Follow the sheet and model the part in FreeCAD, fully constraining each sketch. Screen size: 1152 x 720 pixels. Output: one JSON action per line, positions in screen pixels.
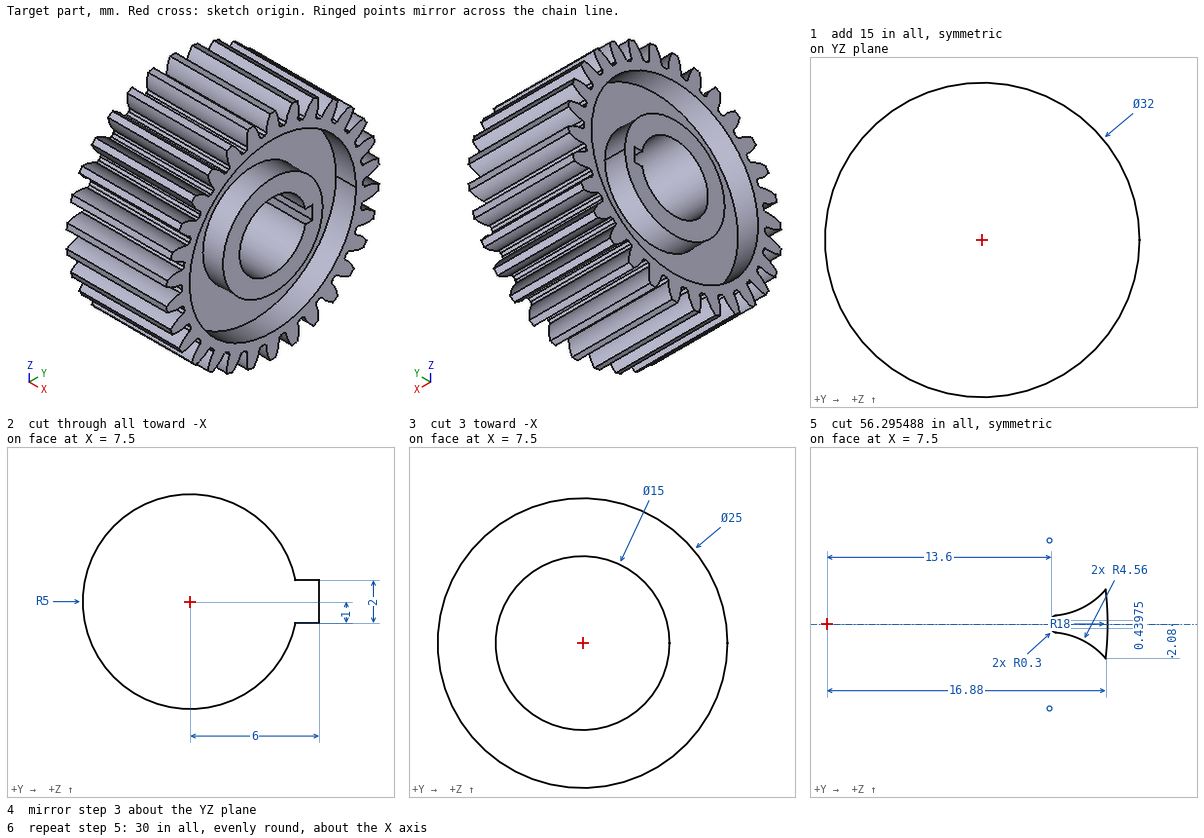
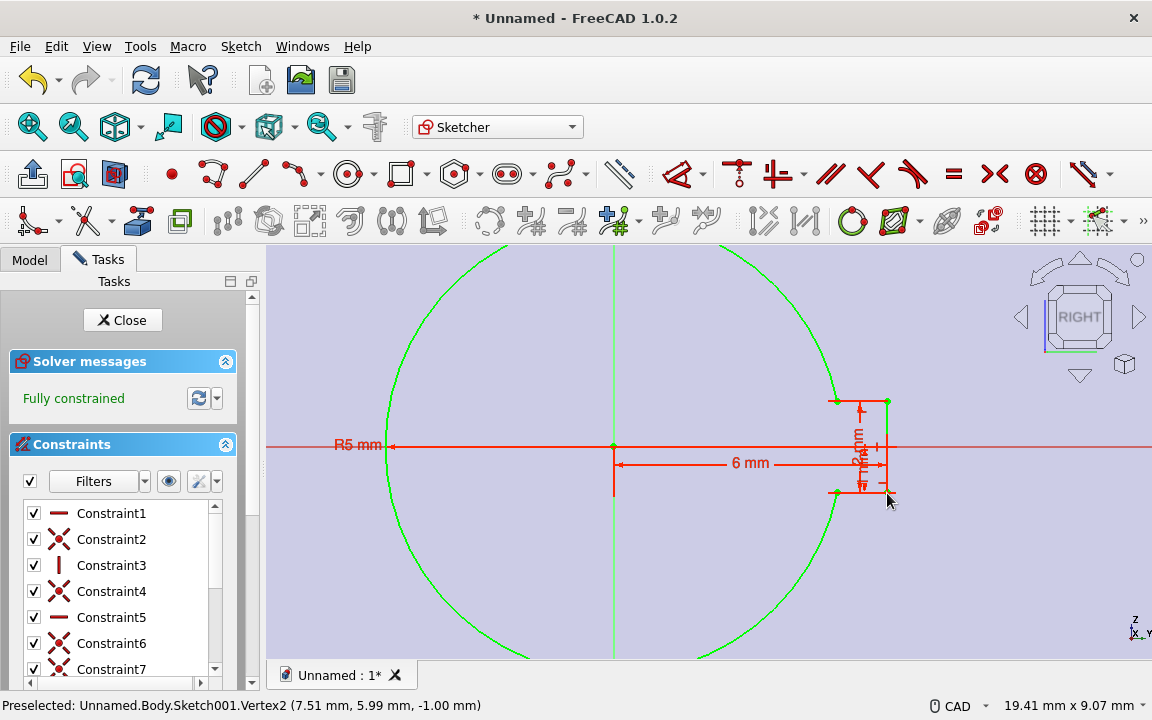
{"action": "left_click", "coordinate": [123, 320]}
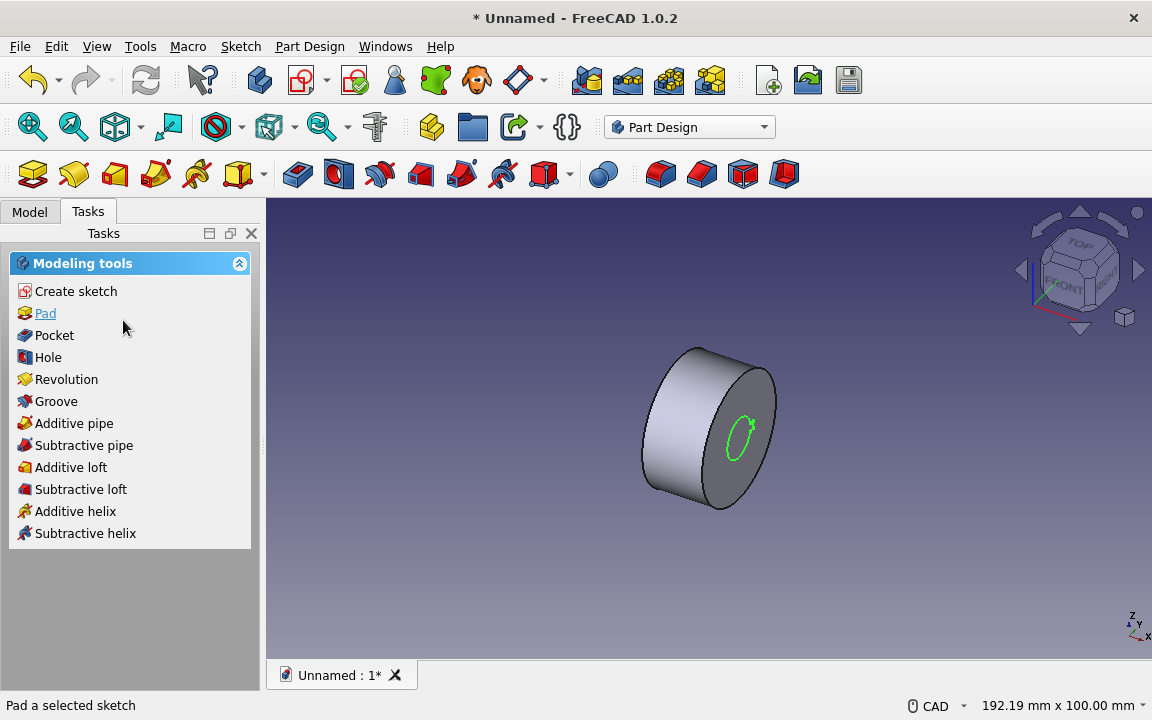
{"action": "left_click", "coordinate": [298, 174]}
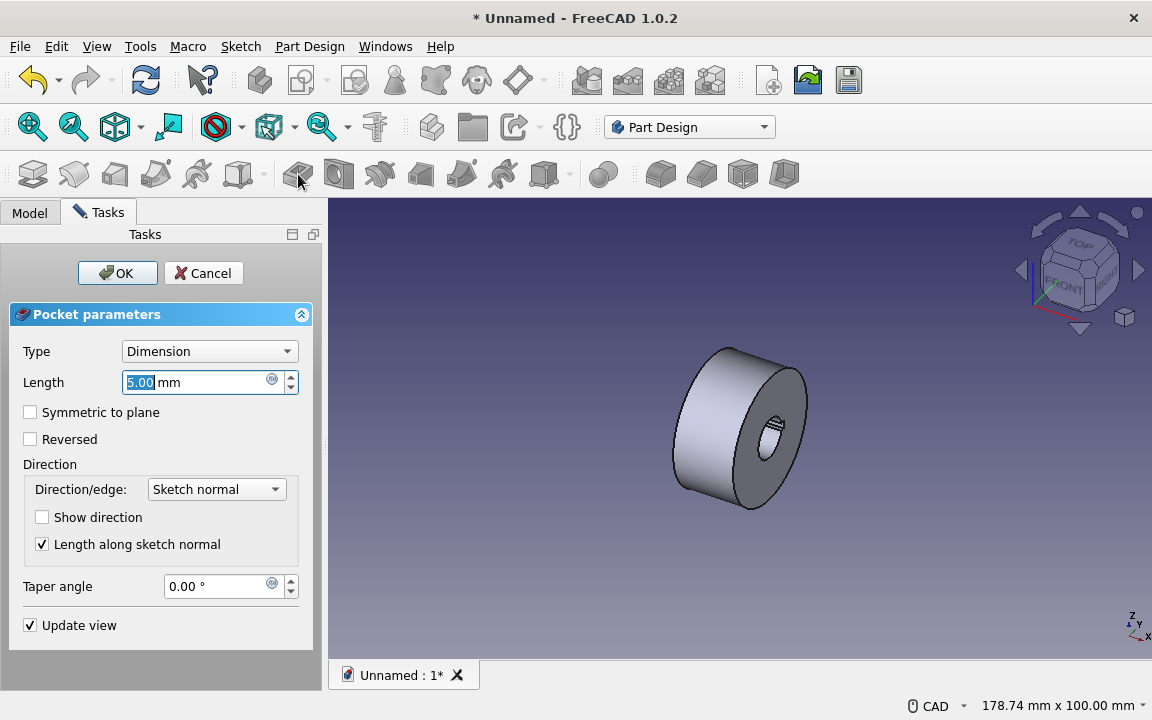
{"action": "left_click", "coordinate": [210, 352]}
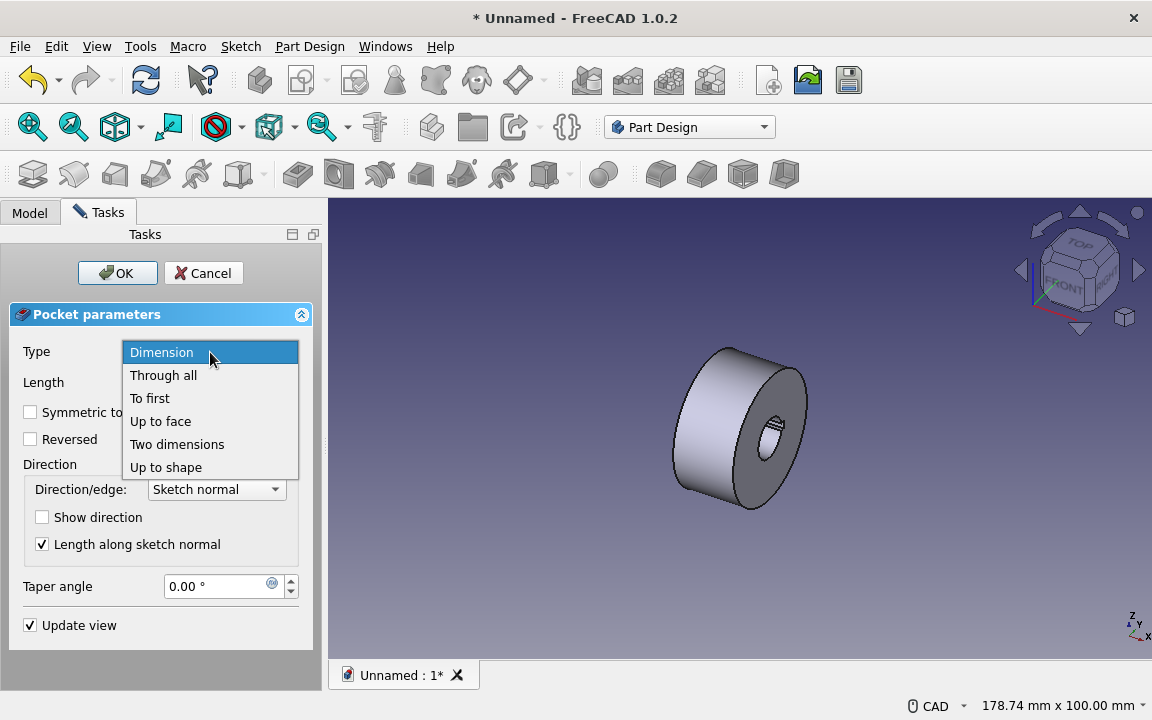
{"action": "left_click", "coordinate": [208, 376]}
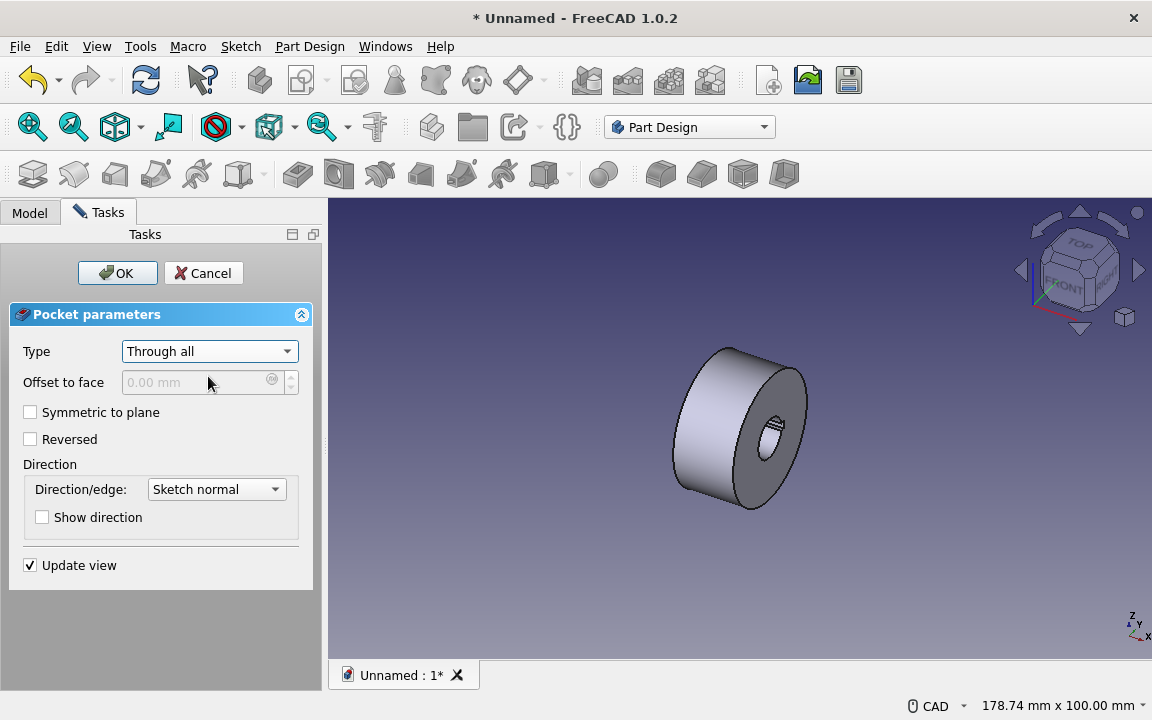
{"action": "left_click", "coordinate": [118, 273]}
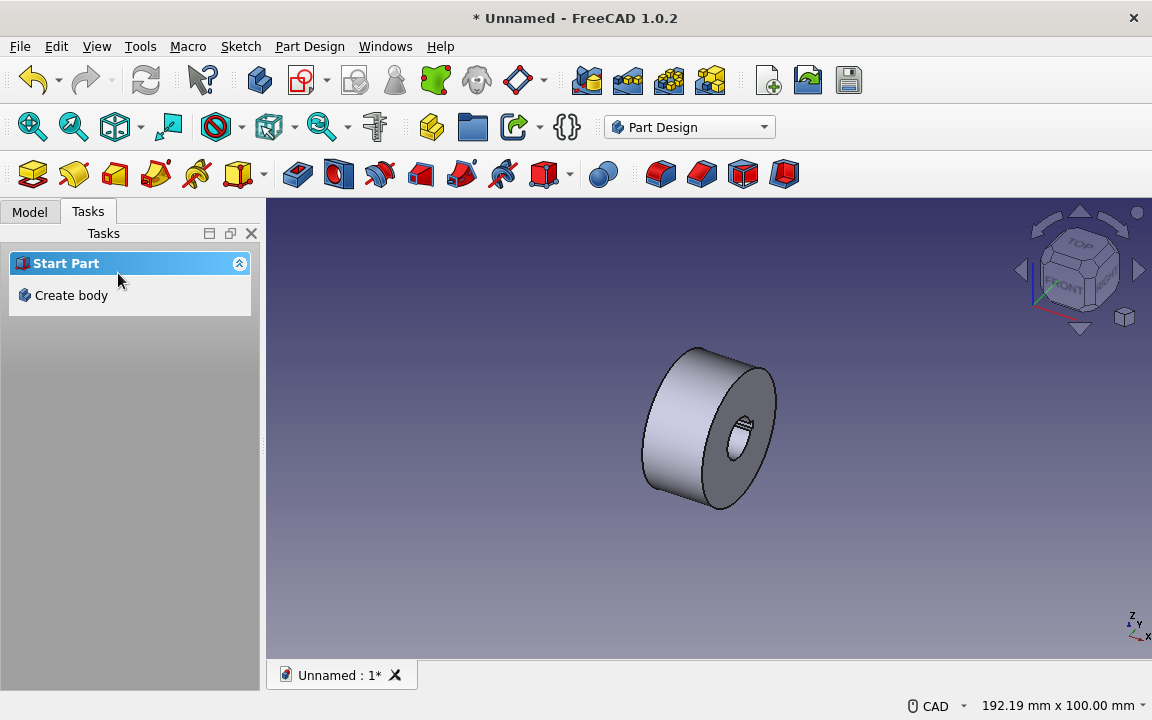
{"action": "left_click", "coordinate": [718, 441]}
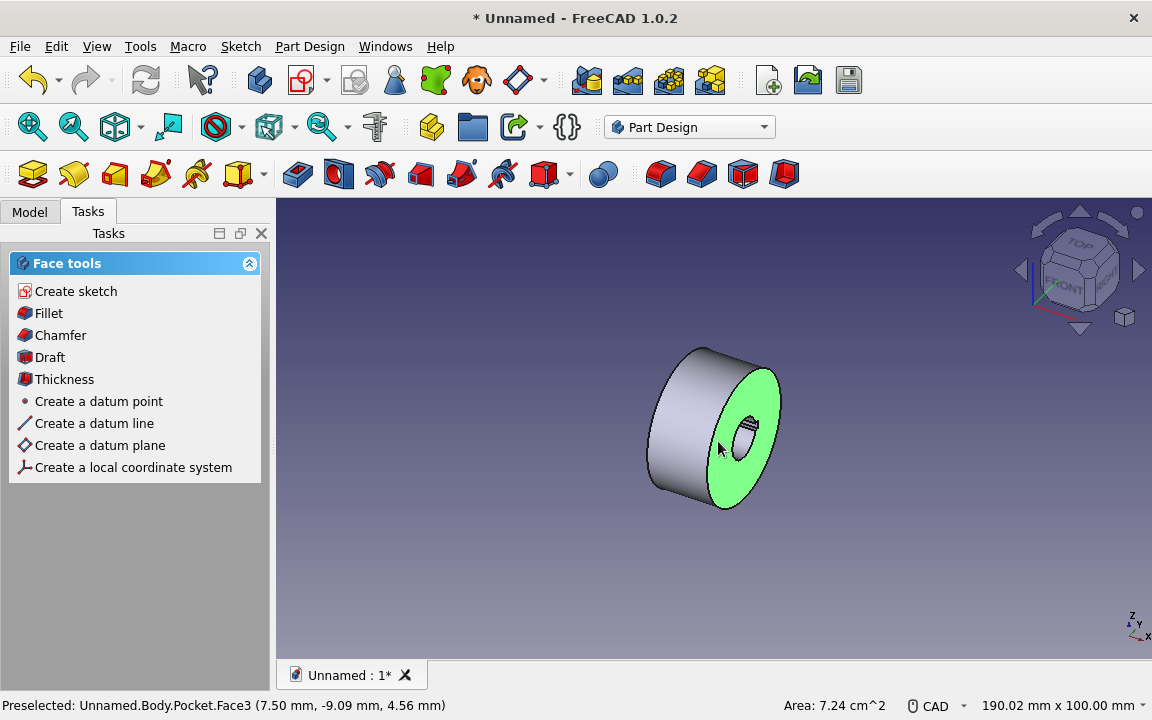
{"action": "left_click", "coordinate": [300, 80]}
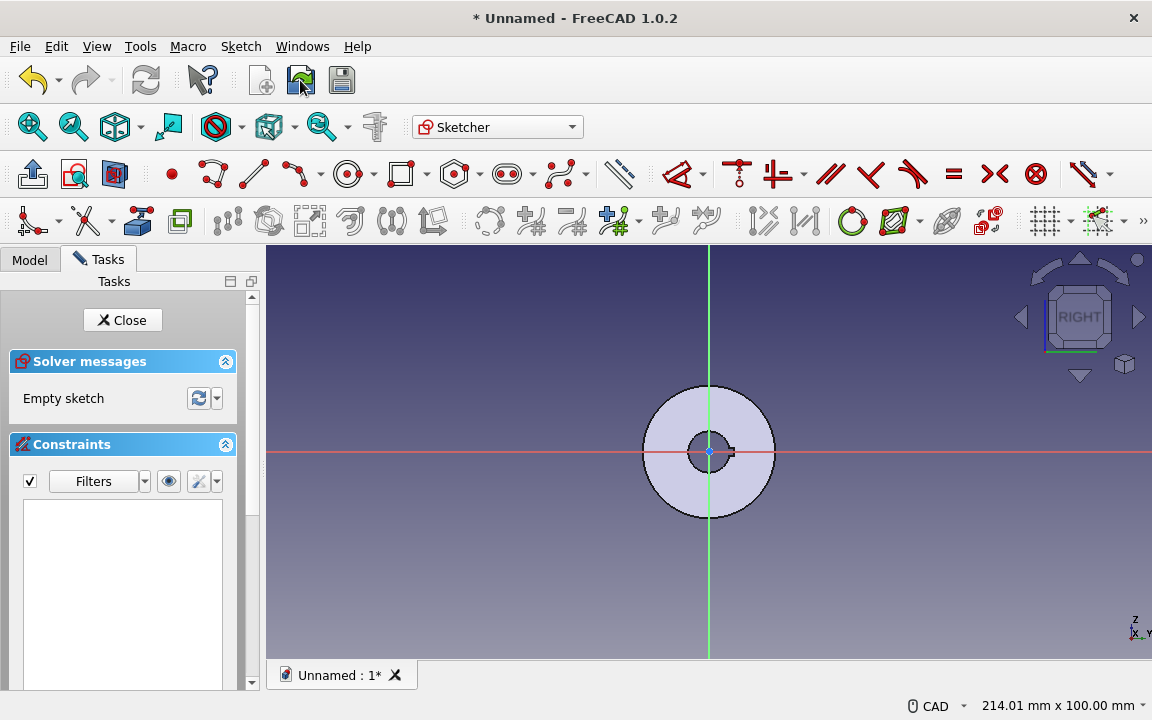
{"action": "scroll", "coordinate": [765, 452], "scroll_direction": "up", "scroll_amount": 4}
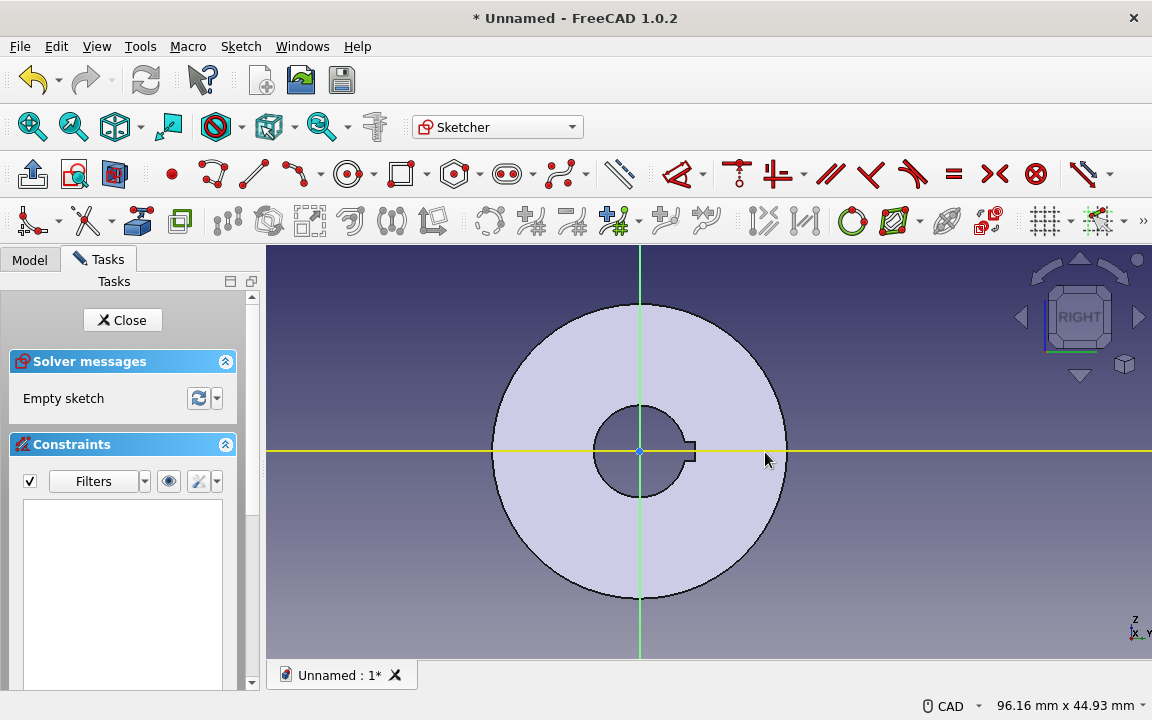
{"action": "key", "text": "g c"}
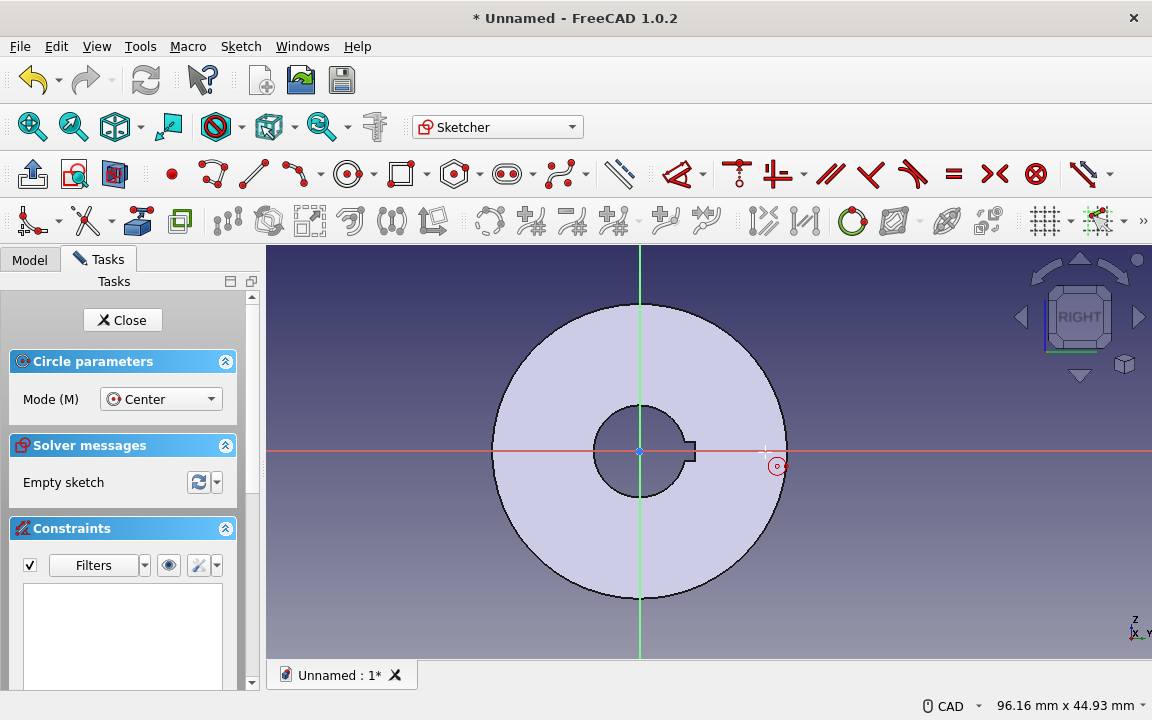
{"action": "left_click", "coordinate": [640, 451]}
{"action": "left_click", "coordinate": [721, 370]}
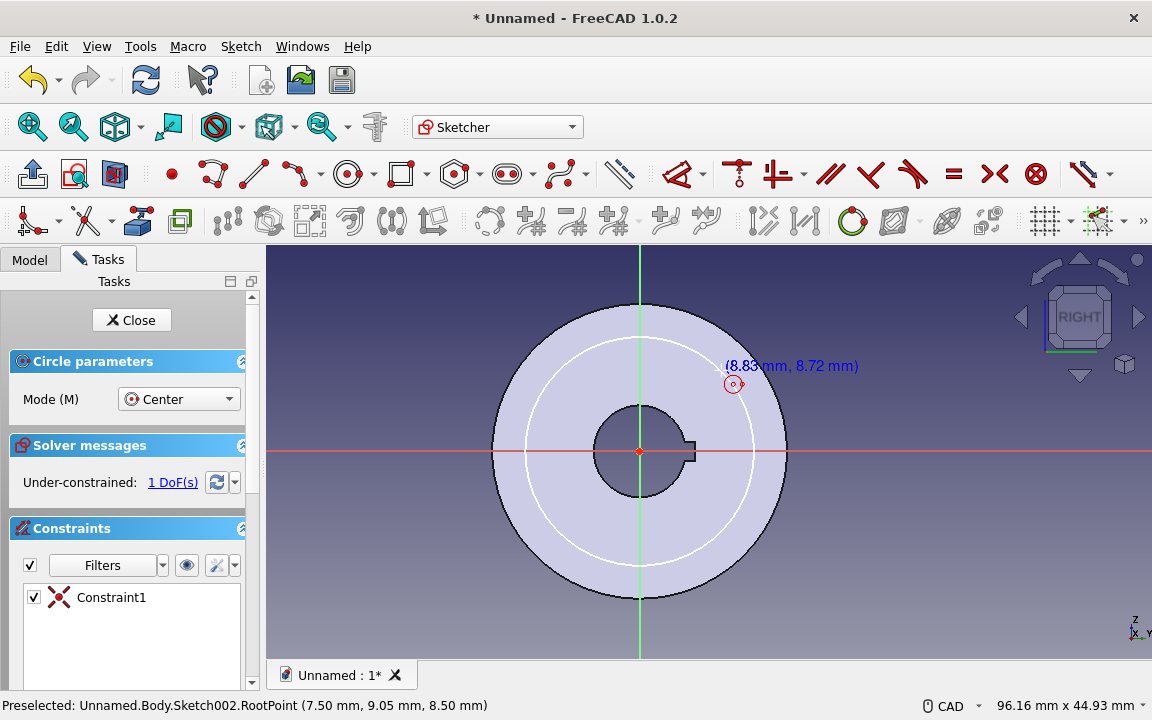
{"action": "left_click", "coordinate": [640, 451]}
{"action": "left_click", "coordinate": [689, 403]}
{"action": "key", "text": "Escape"}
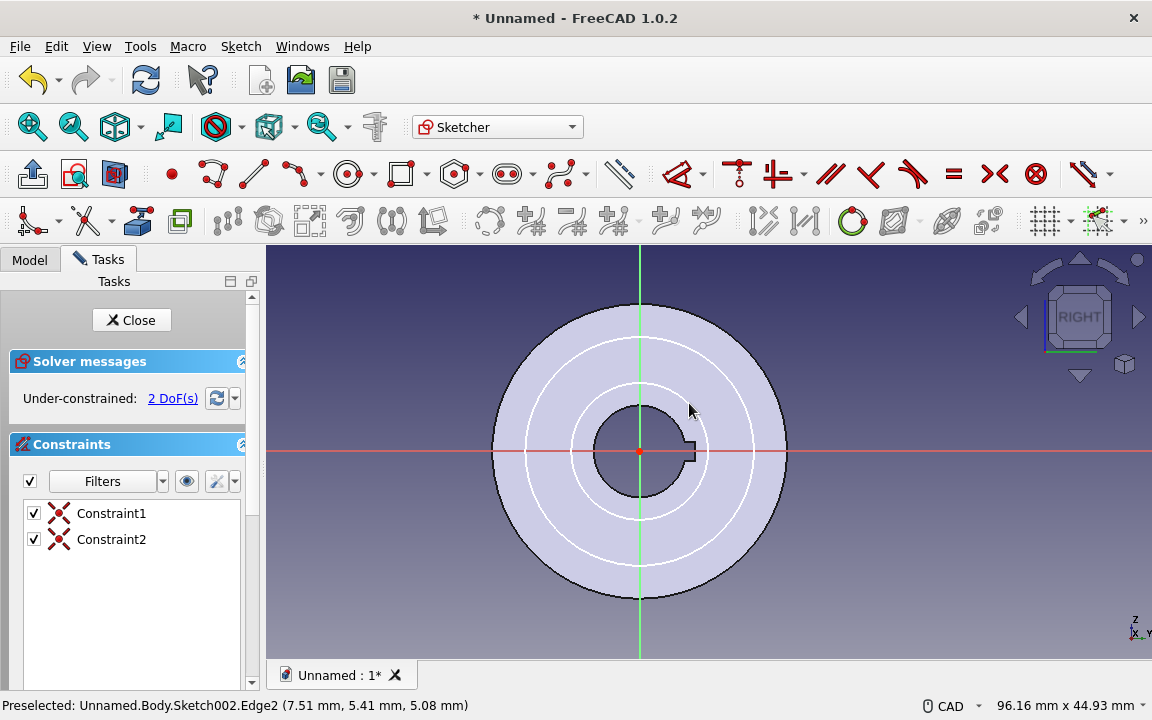
{"action": "left_click", "coordinate": [720, 370]}